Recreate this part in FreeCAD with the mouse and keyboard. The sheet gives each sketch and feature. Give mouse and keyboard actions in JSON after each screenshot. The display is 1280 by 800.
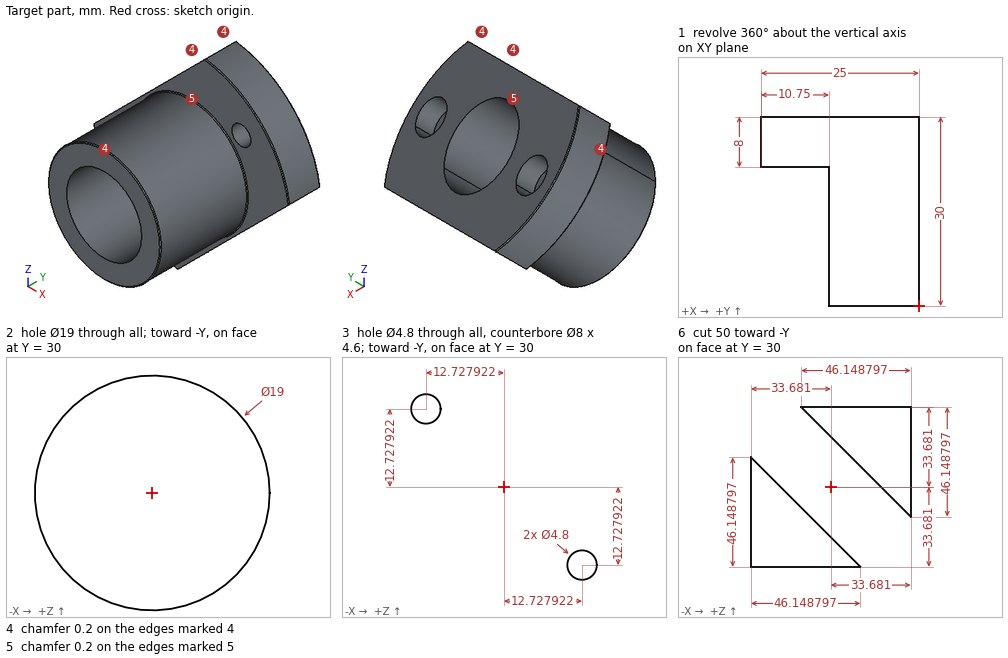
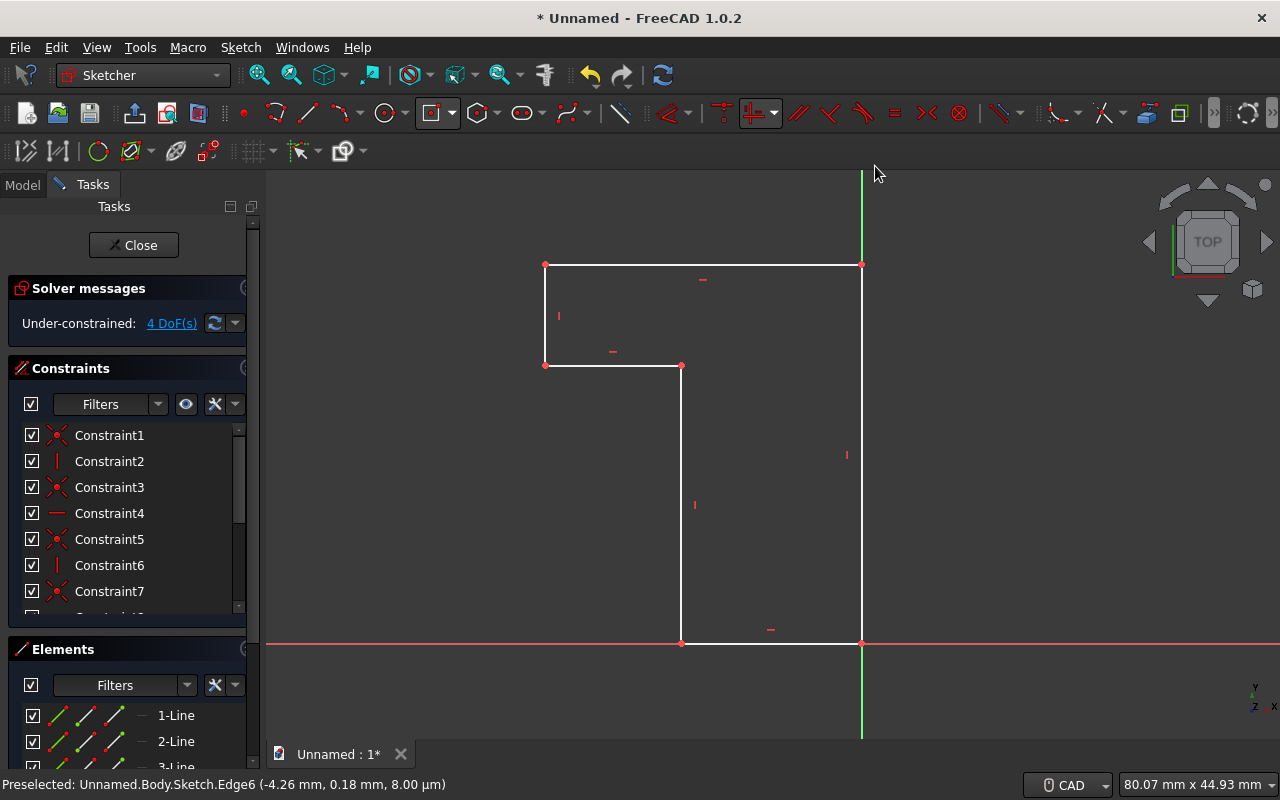
{"action": "left_click", "coordinate": [668, 114]}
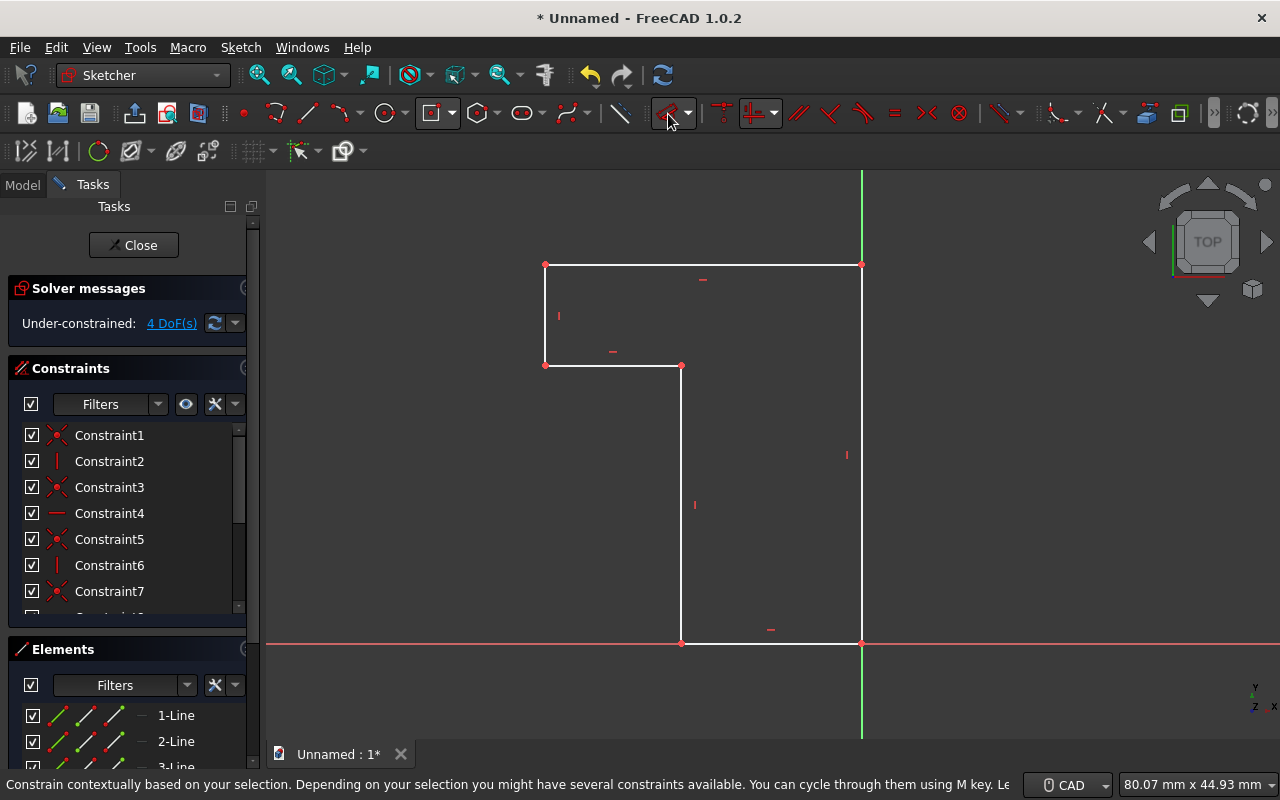
{"action": "left_click", "coordinate": [545, 295]}
{"action": "left_click", "coordinate": [511, 315]}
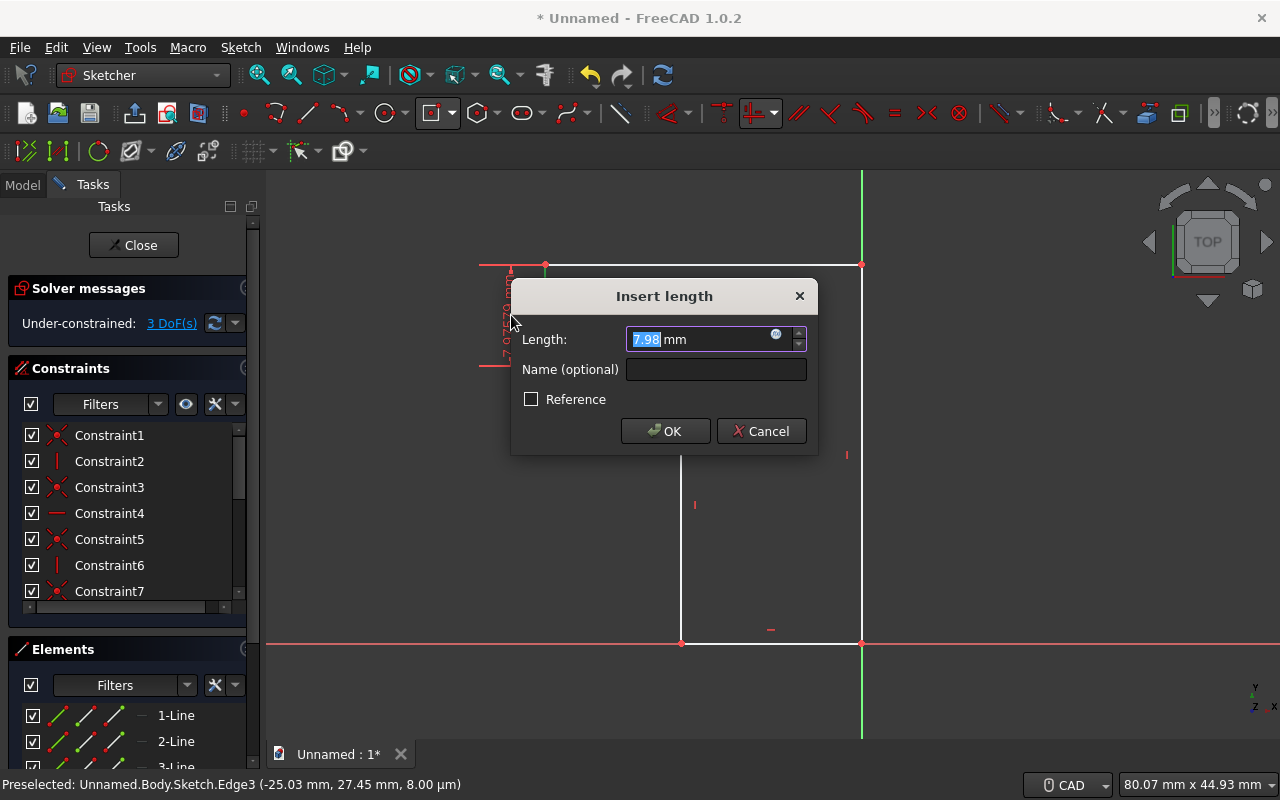
{"action": "type", "text": "8"}
{"action": "key", "text": "Return"}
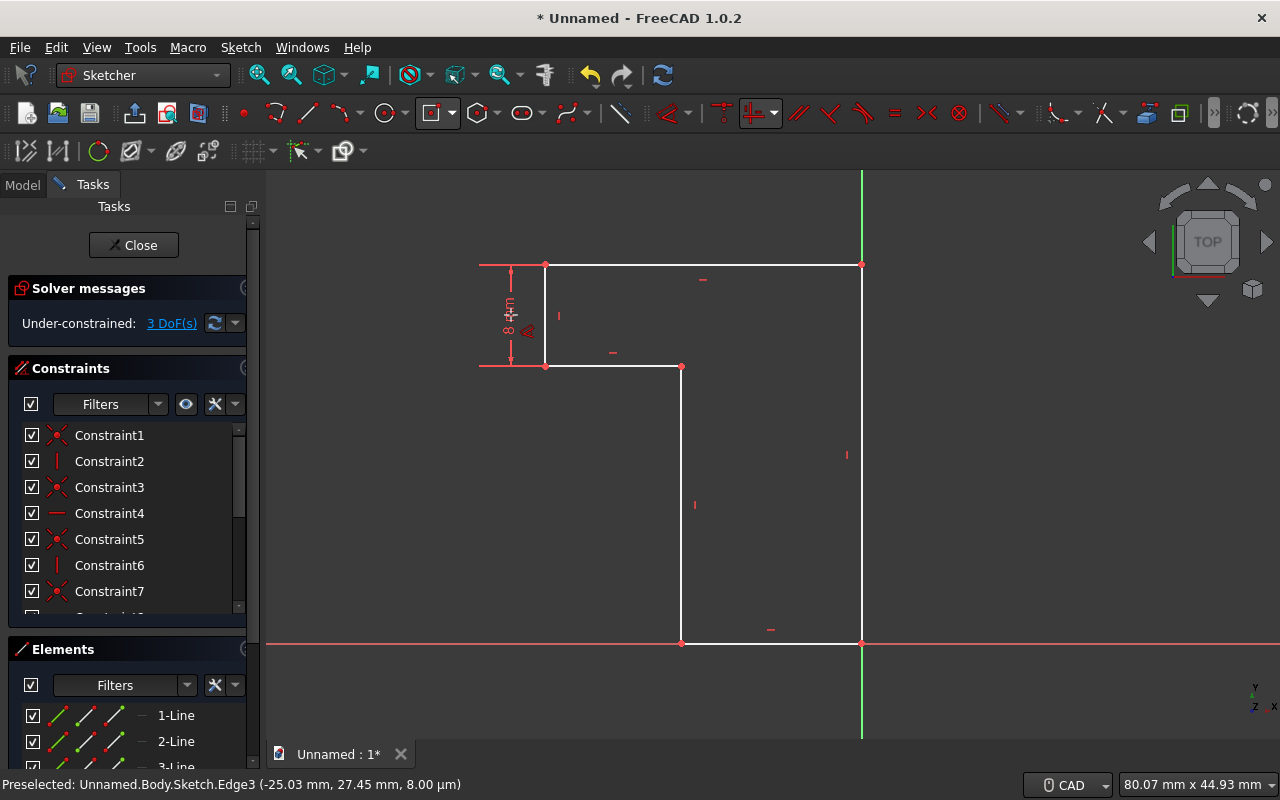
{"action": "left_click", "coordinate": [862, 530]}
{"action": "left_click", "coordinate": [896, 454]}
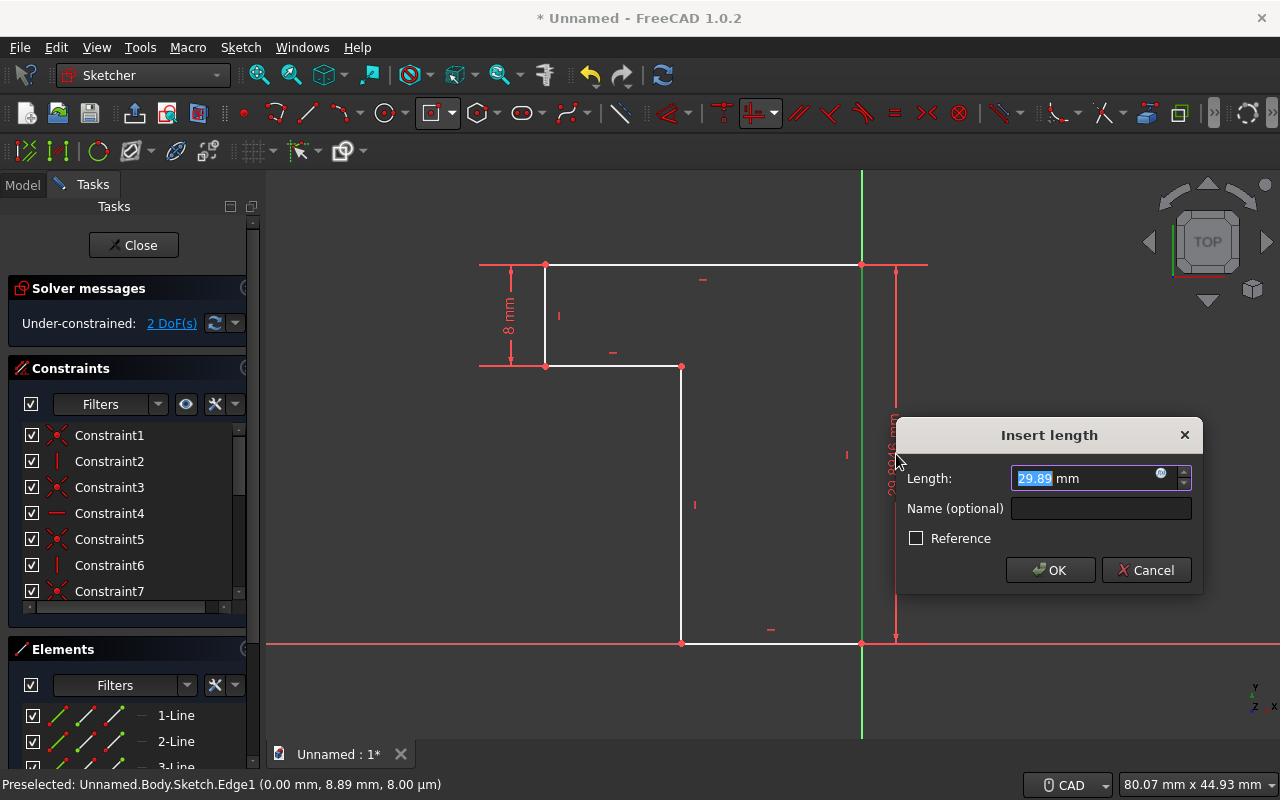
{"action": "type", "text": "30"}
{"action": "key", "text": "Return"}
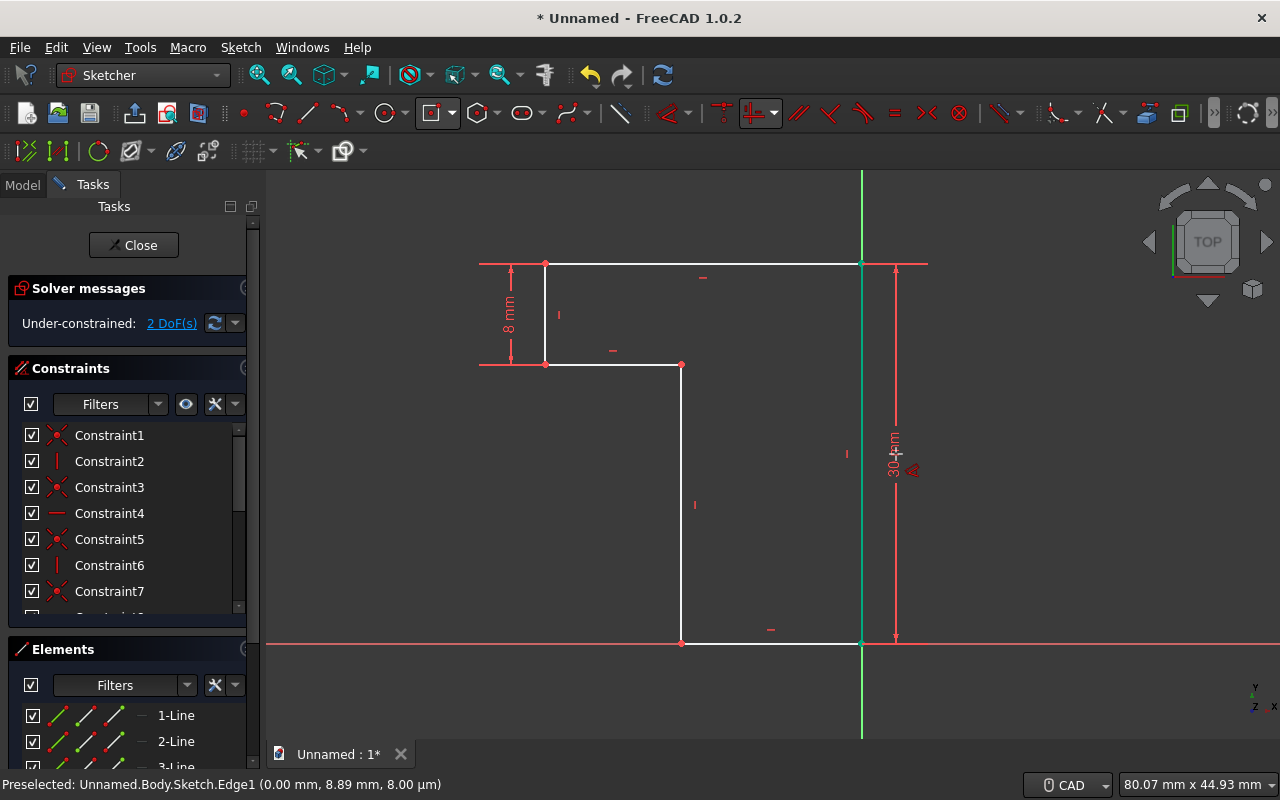
{"action": "left_click", "coordinate": [767, 264]}
{"action": "left_click", "coordinate": [703, 230]}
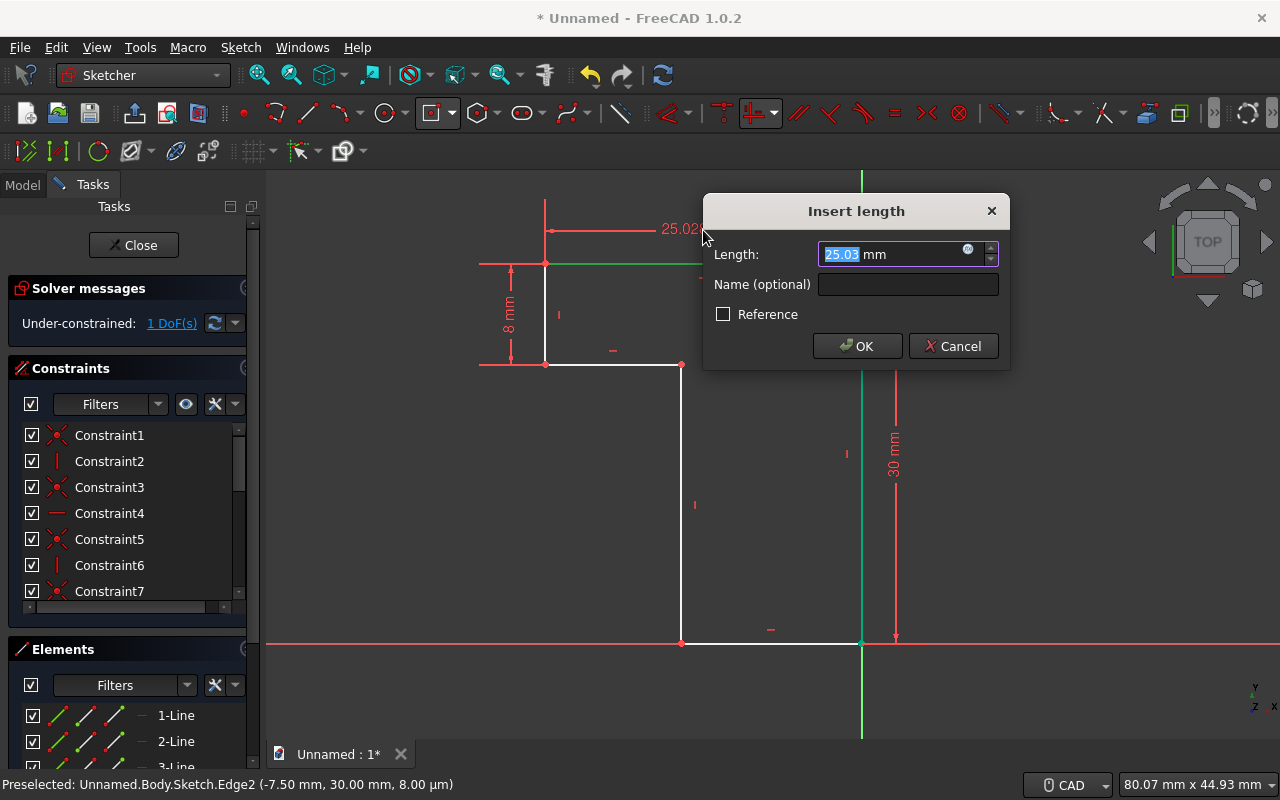
{"action": "type", "text": "25"}
{"action": "key", "text": "Return"}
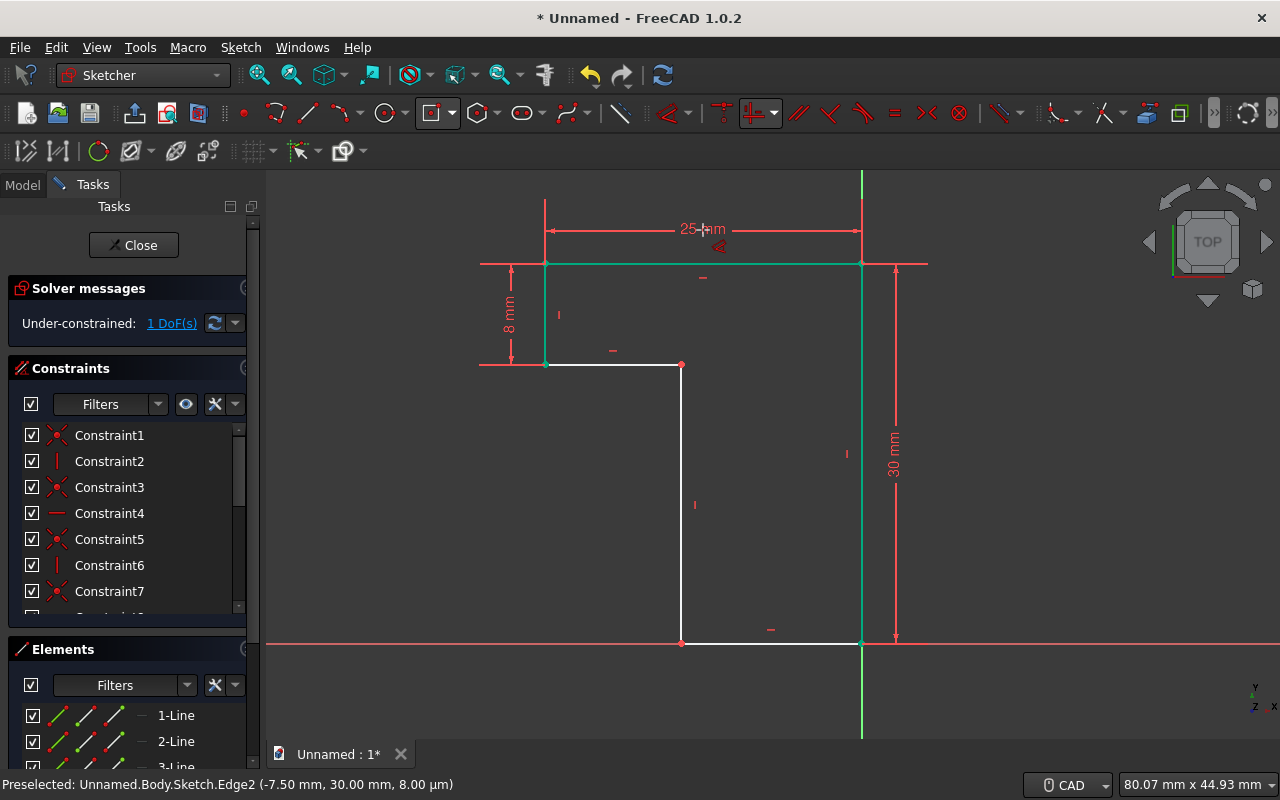
{"action": "left_click", "coordinate": [586, 365]}
{"action": "left_click", "coordinate": [613, 331]}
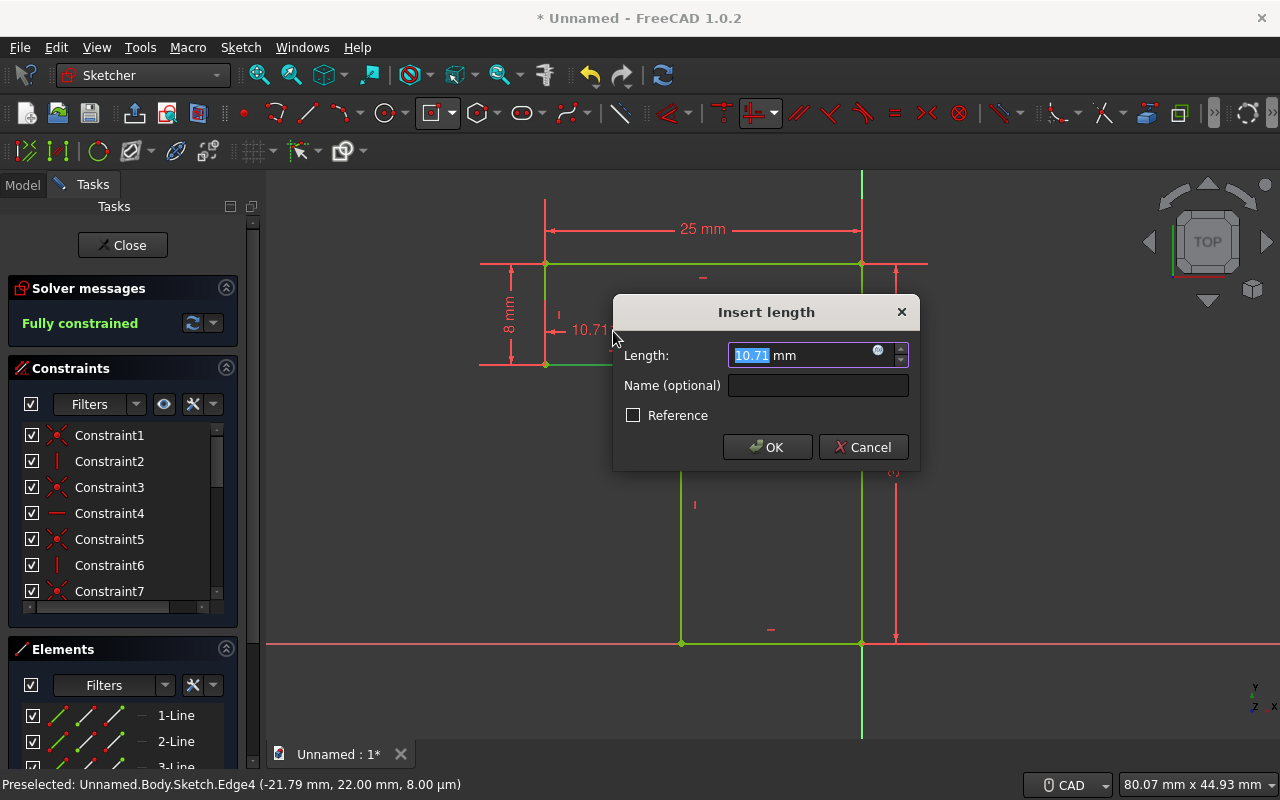
{"action": "type", "text": "10.75"}
{"action": "key", "text": "Return"}
{"action": "key", "text": "Escape"}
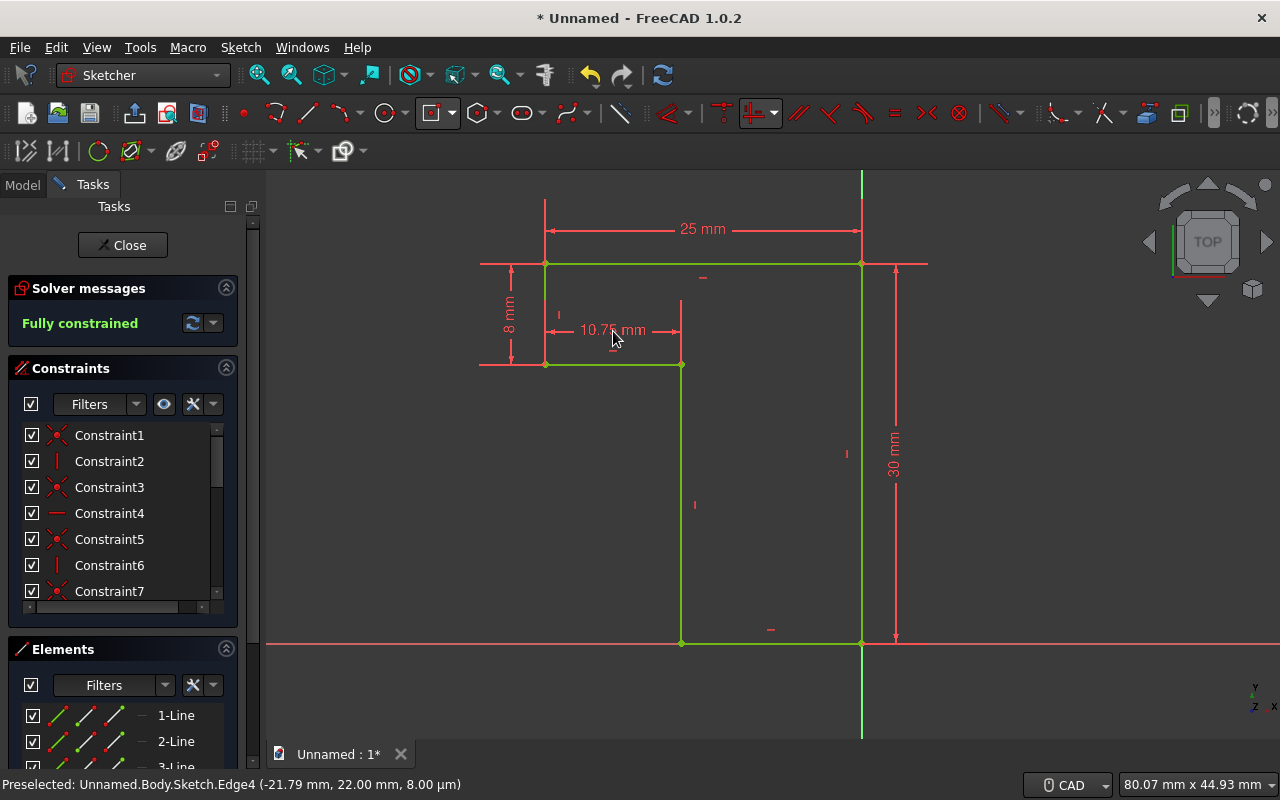
{"action": "left_click", "coordinate": [123, 245]}